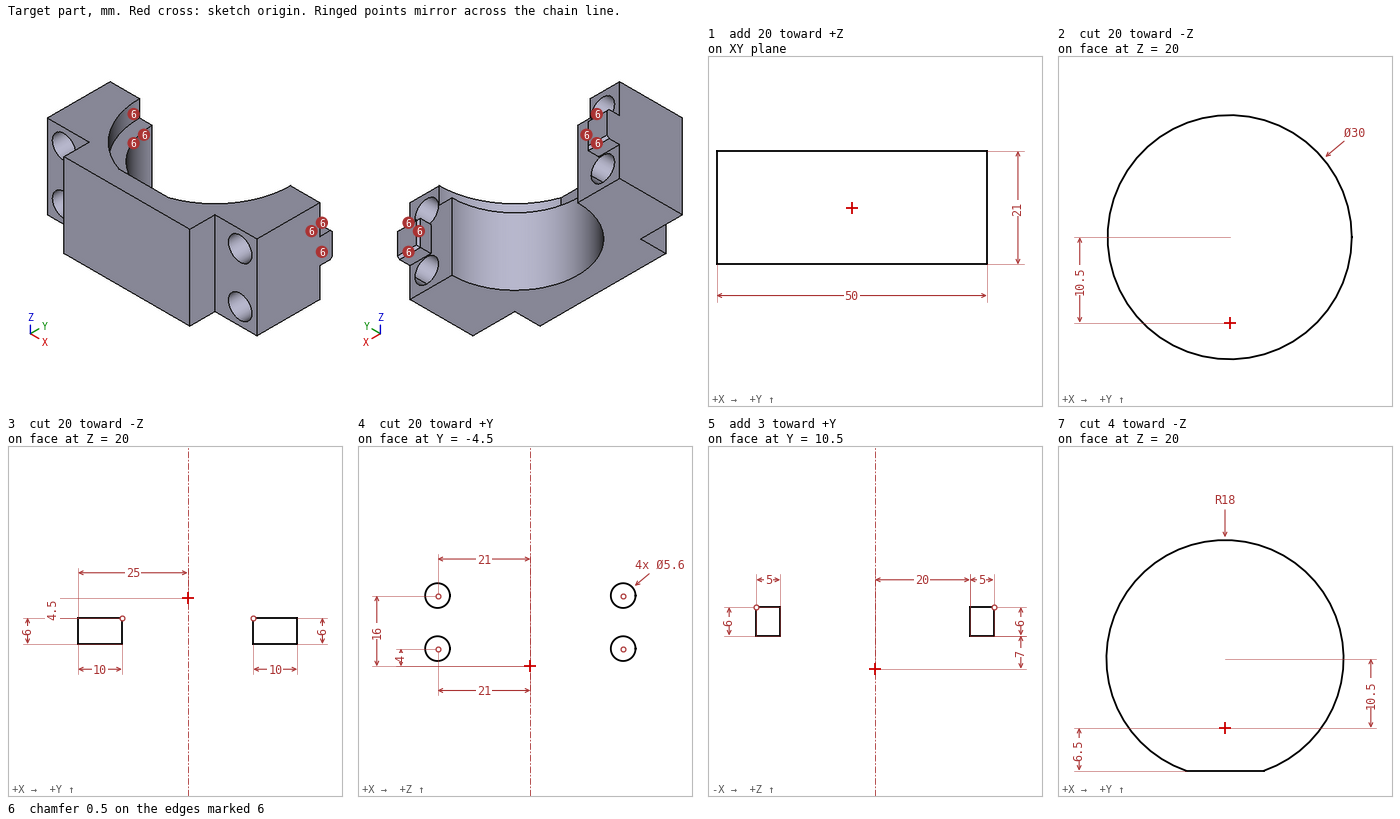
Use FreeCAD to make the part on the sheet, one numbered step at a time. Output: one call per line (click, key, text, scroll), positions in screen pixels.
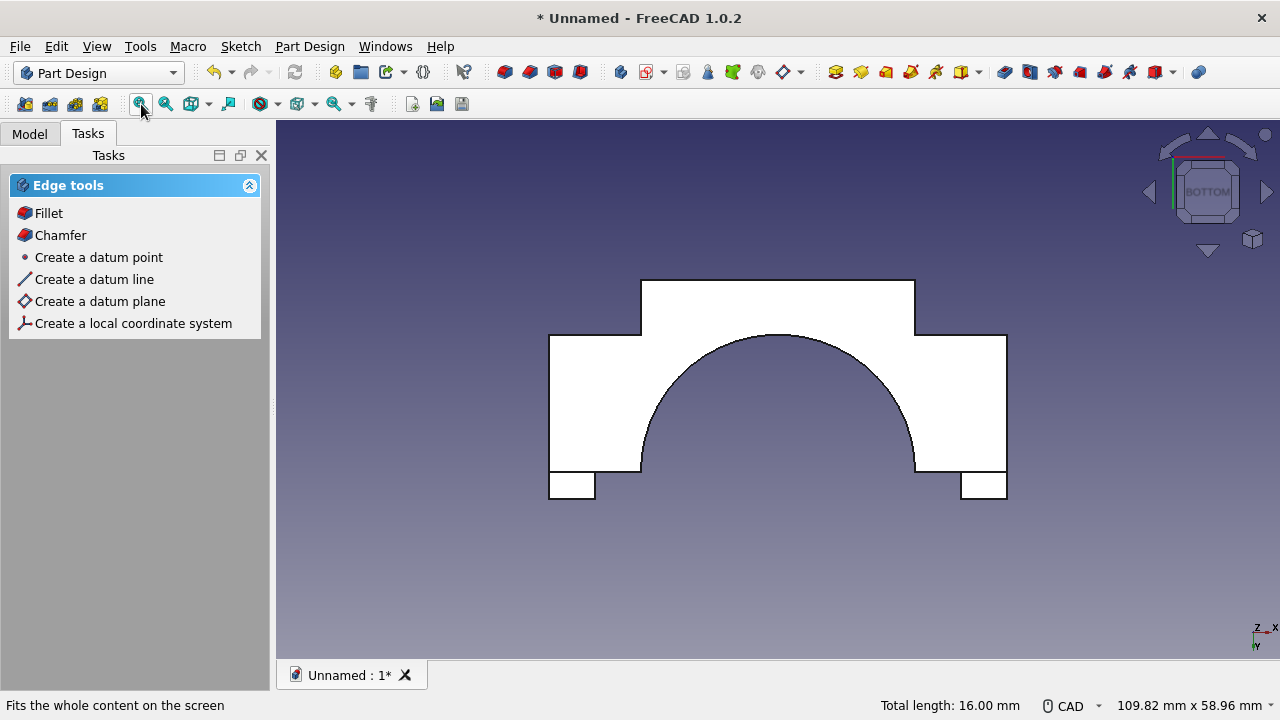
click(572, 498, ctrl)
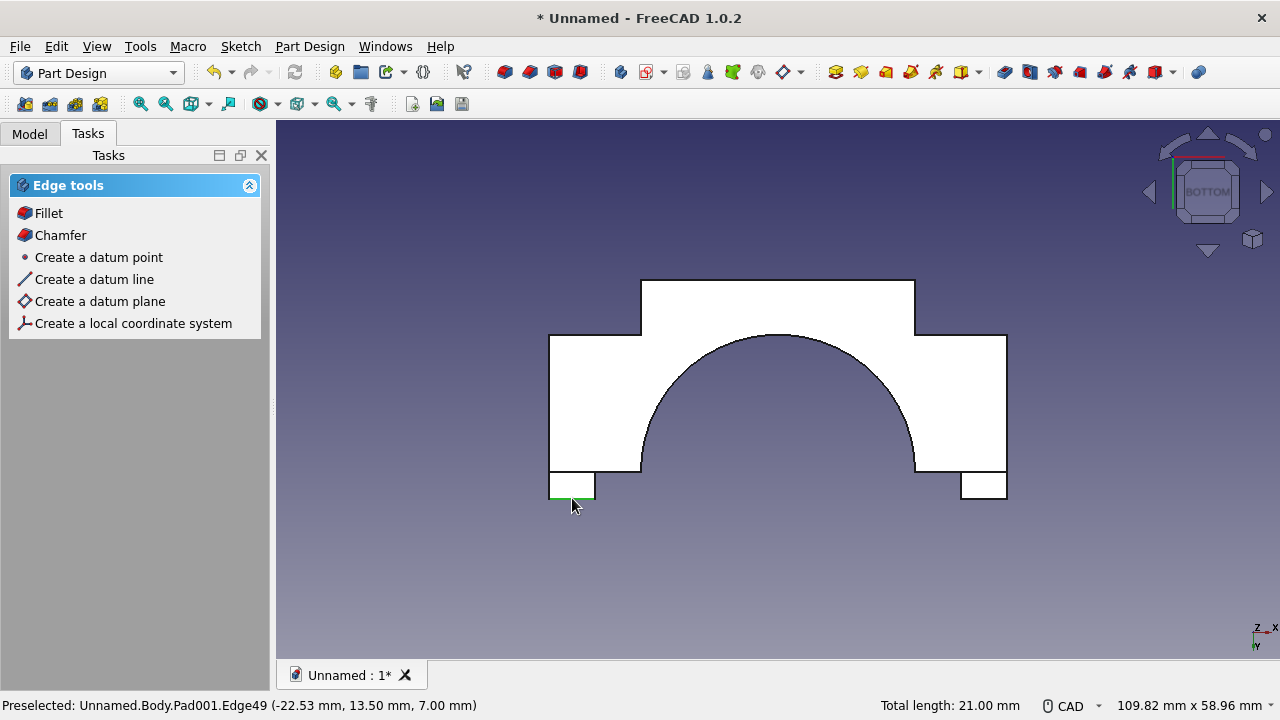
click(984, 498, ctrl)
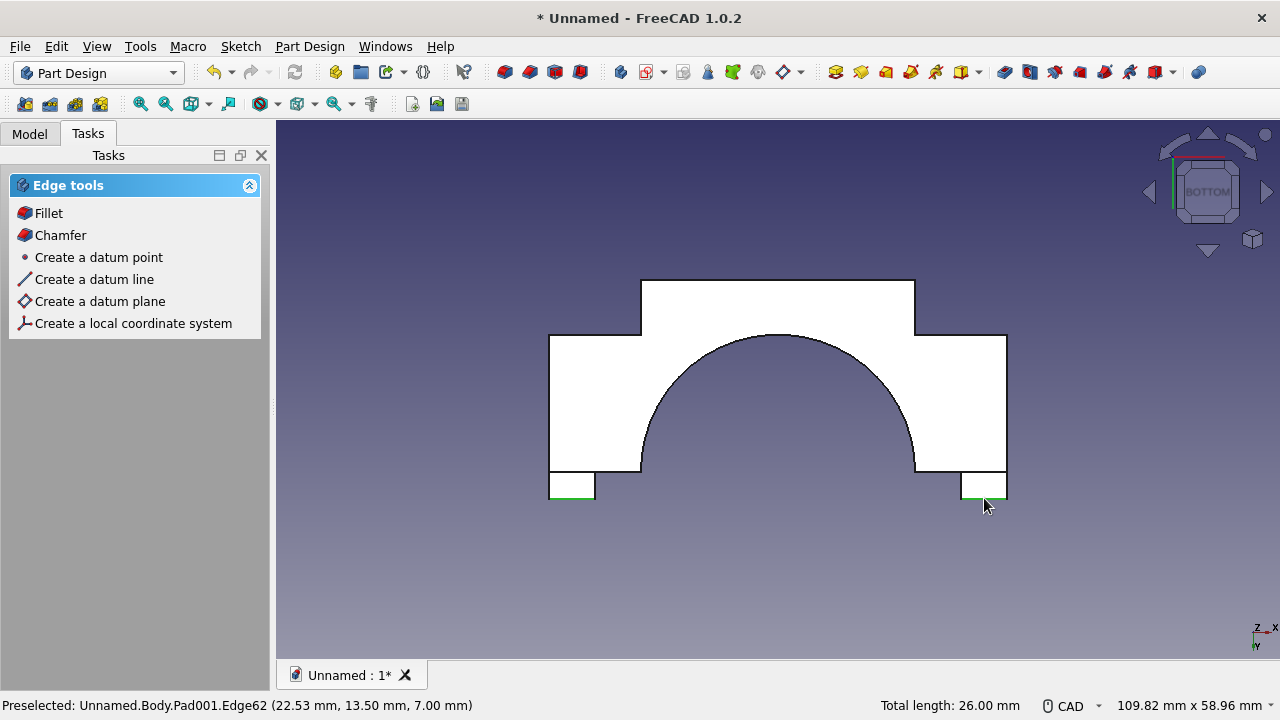
key(4)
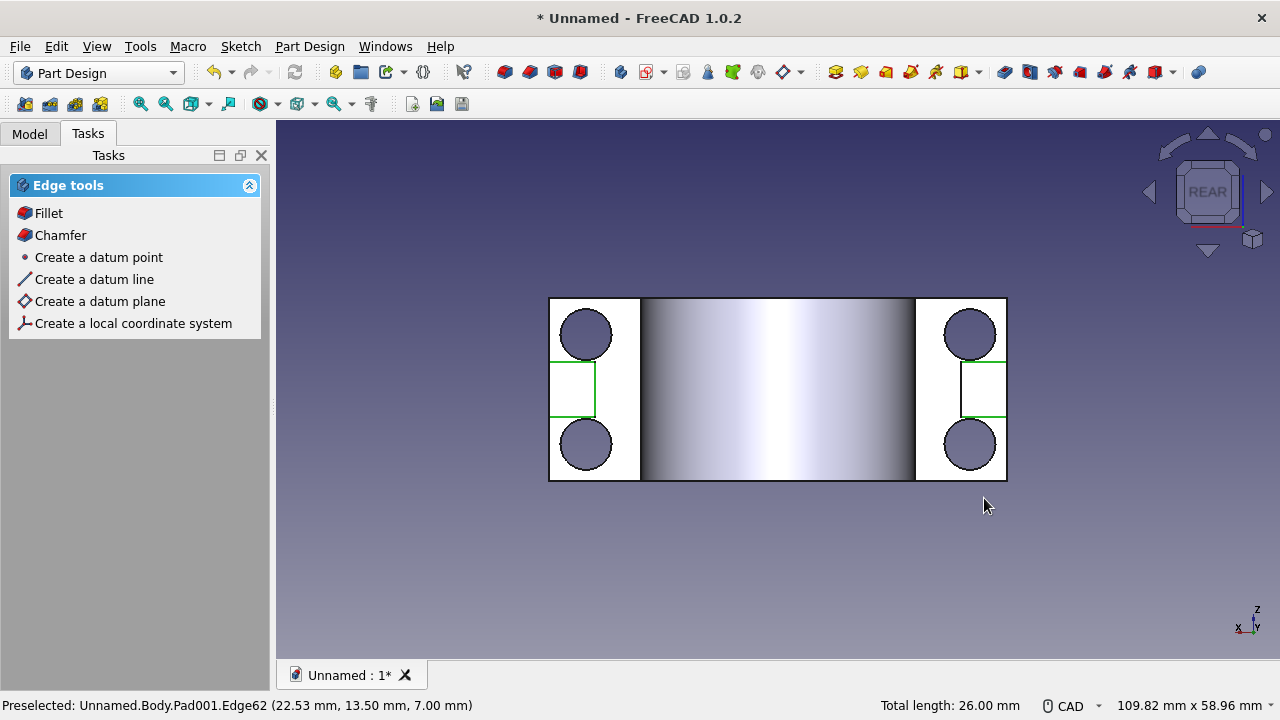
click(961, 388, ctrl)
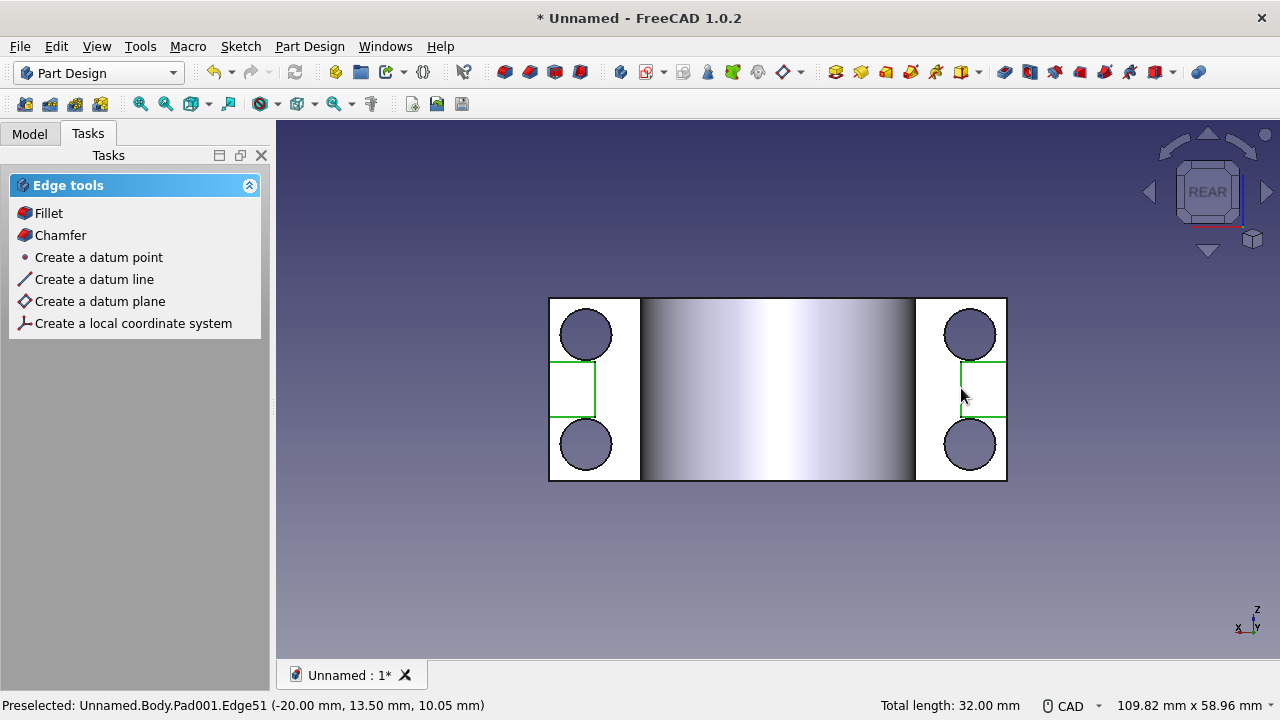
click(530, 72)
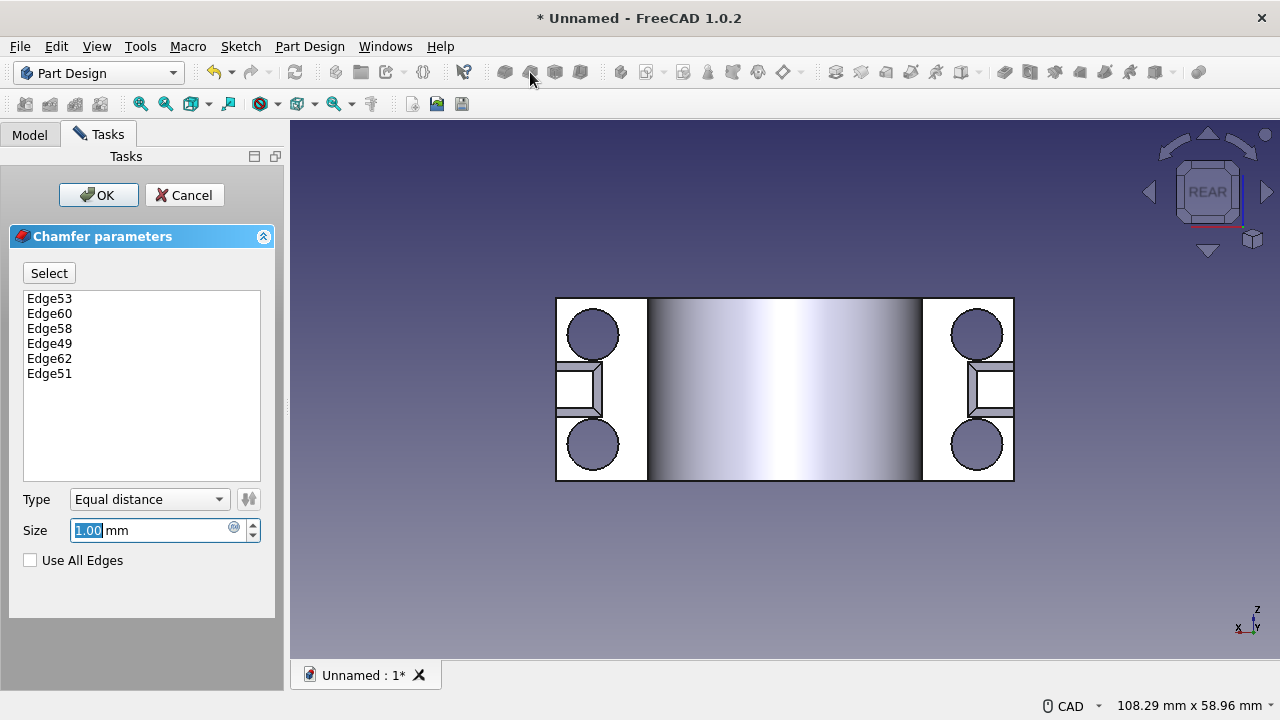
text(0.5)
key(Tab)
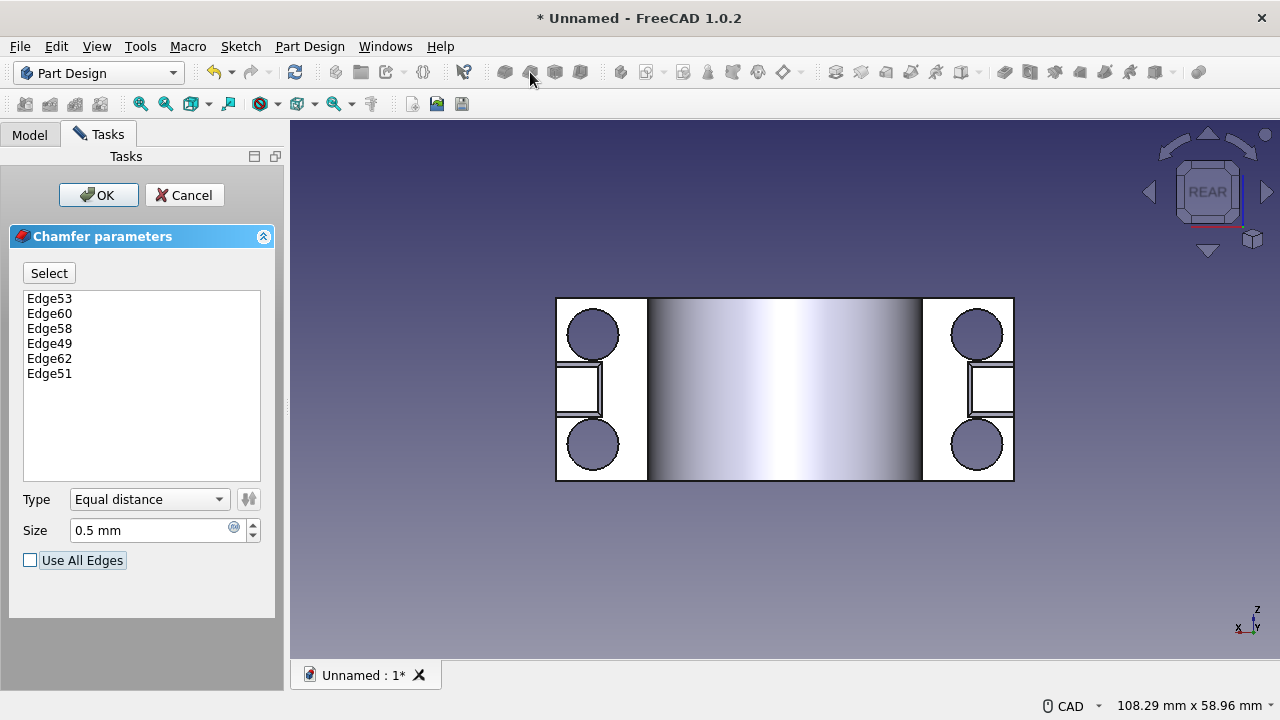
click(99, 195)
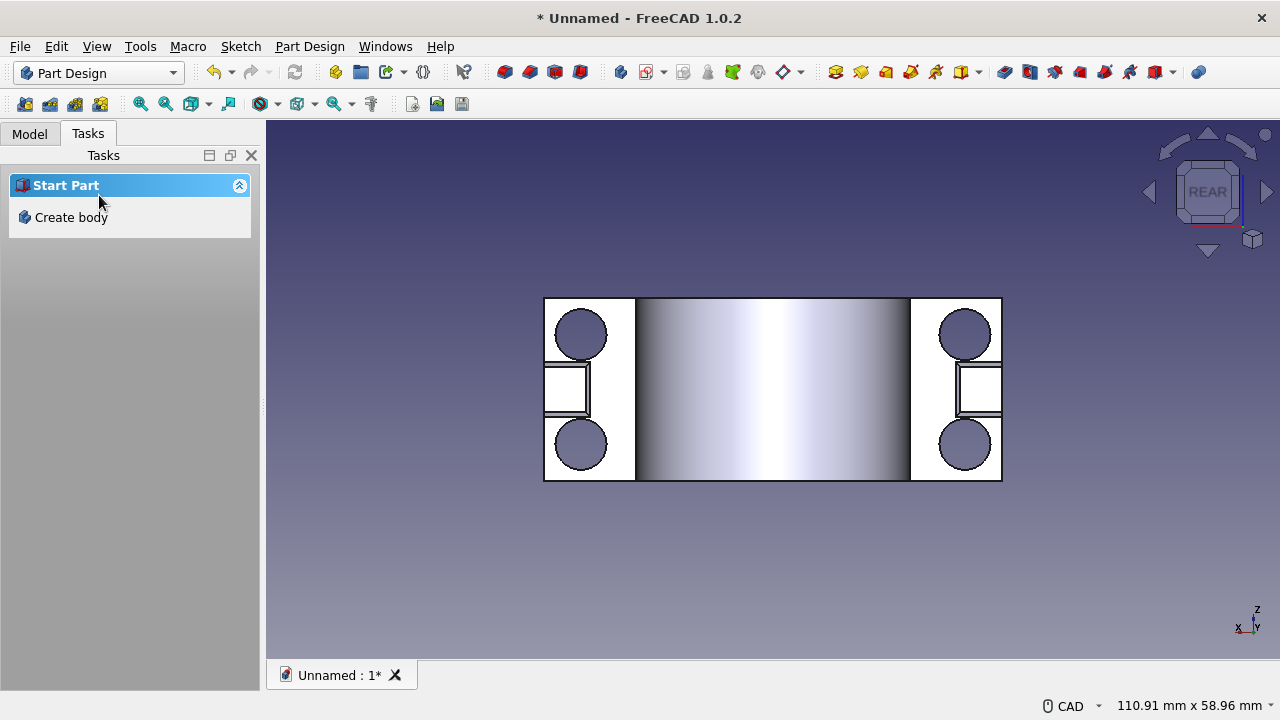
key(0)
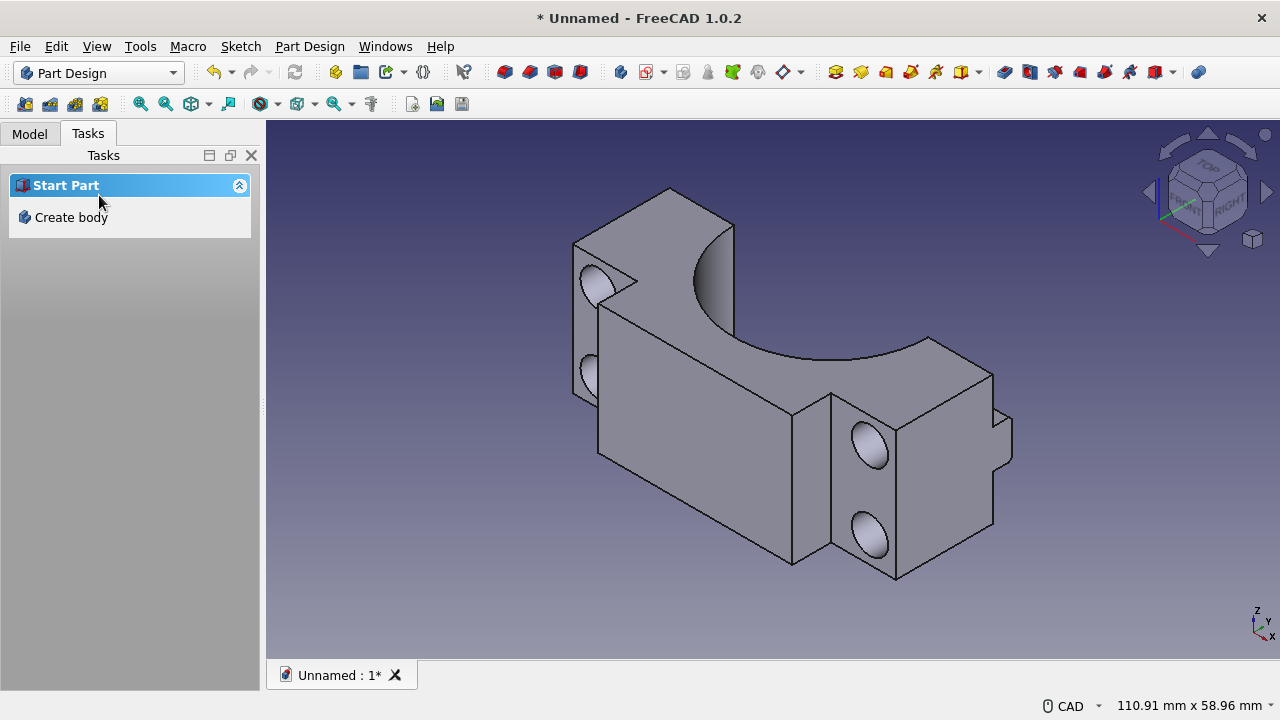
click(664, 217)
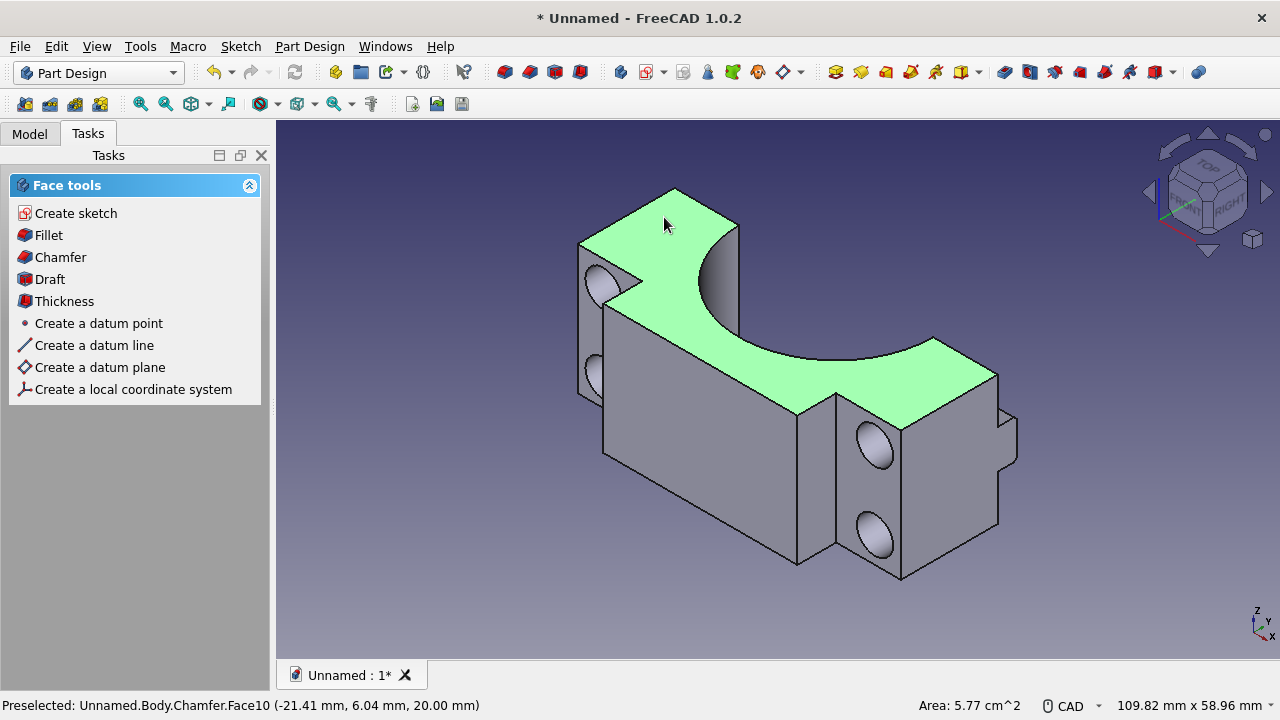
click(646, 72)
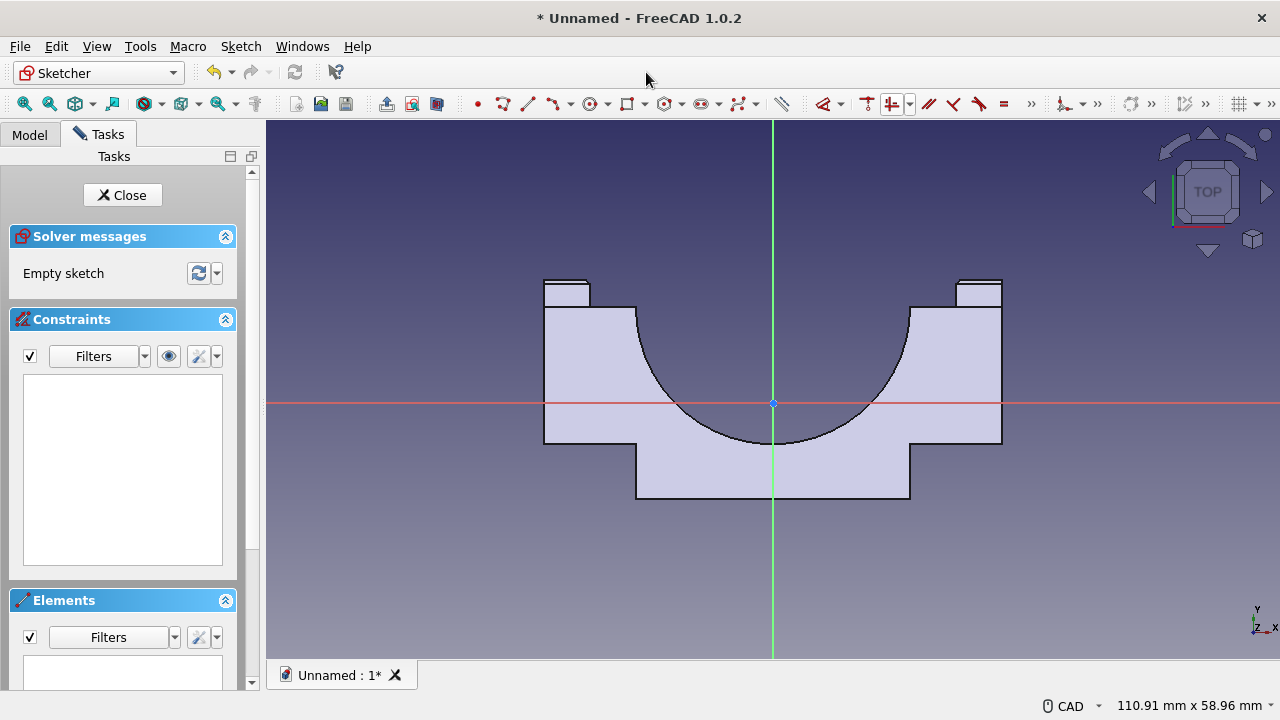
scroll(395, 631, down, 1)